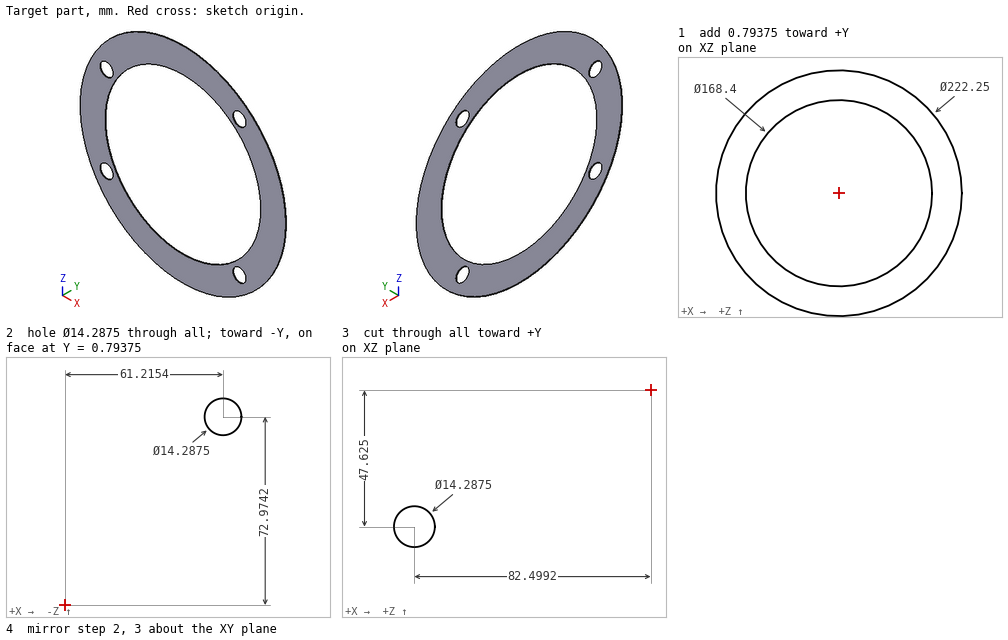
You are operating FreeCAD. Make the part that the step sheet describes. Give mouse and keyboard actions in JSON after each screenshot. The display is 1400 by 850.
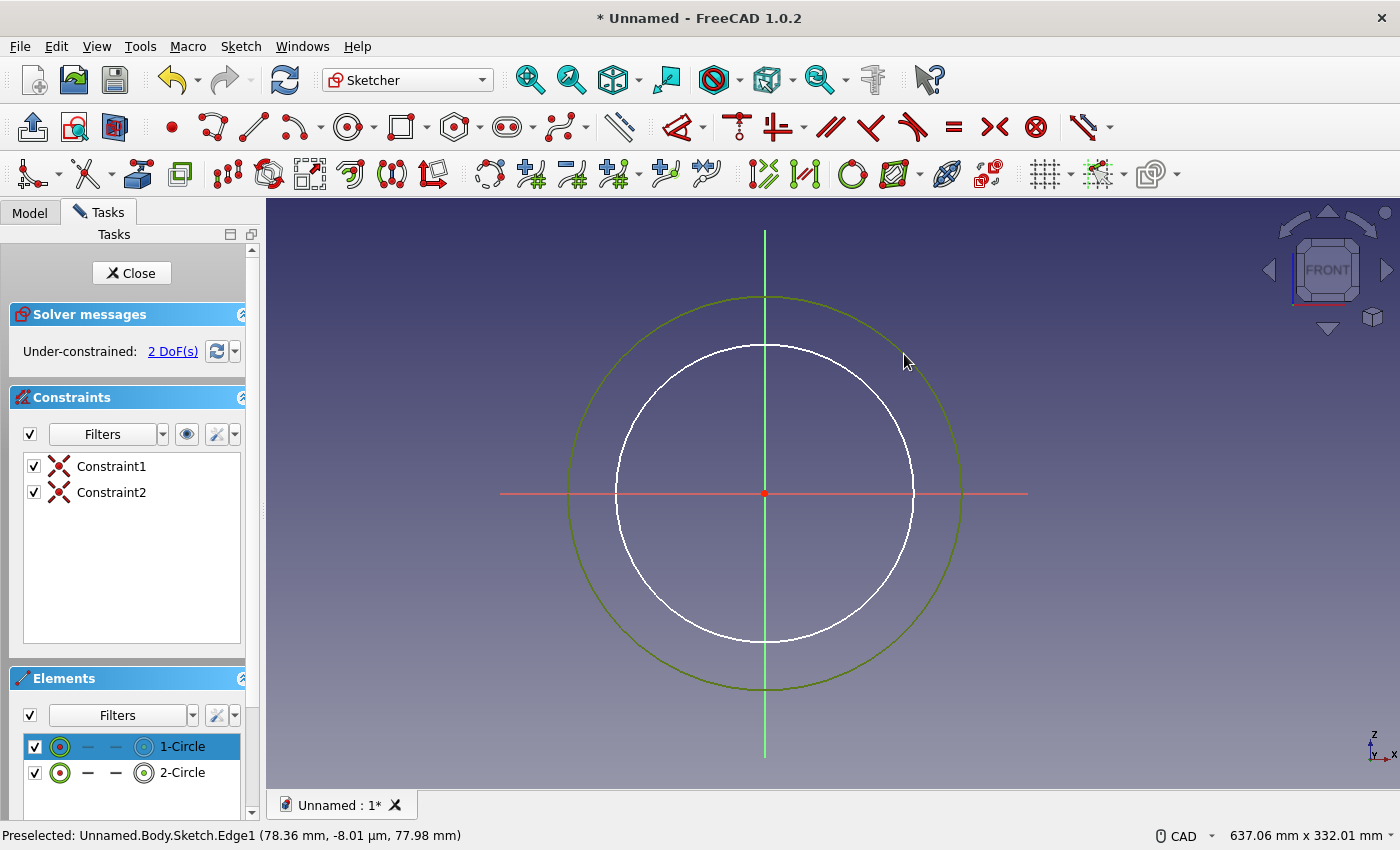
{"action": "left_click", "coordinate": [702, 128]}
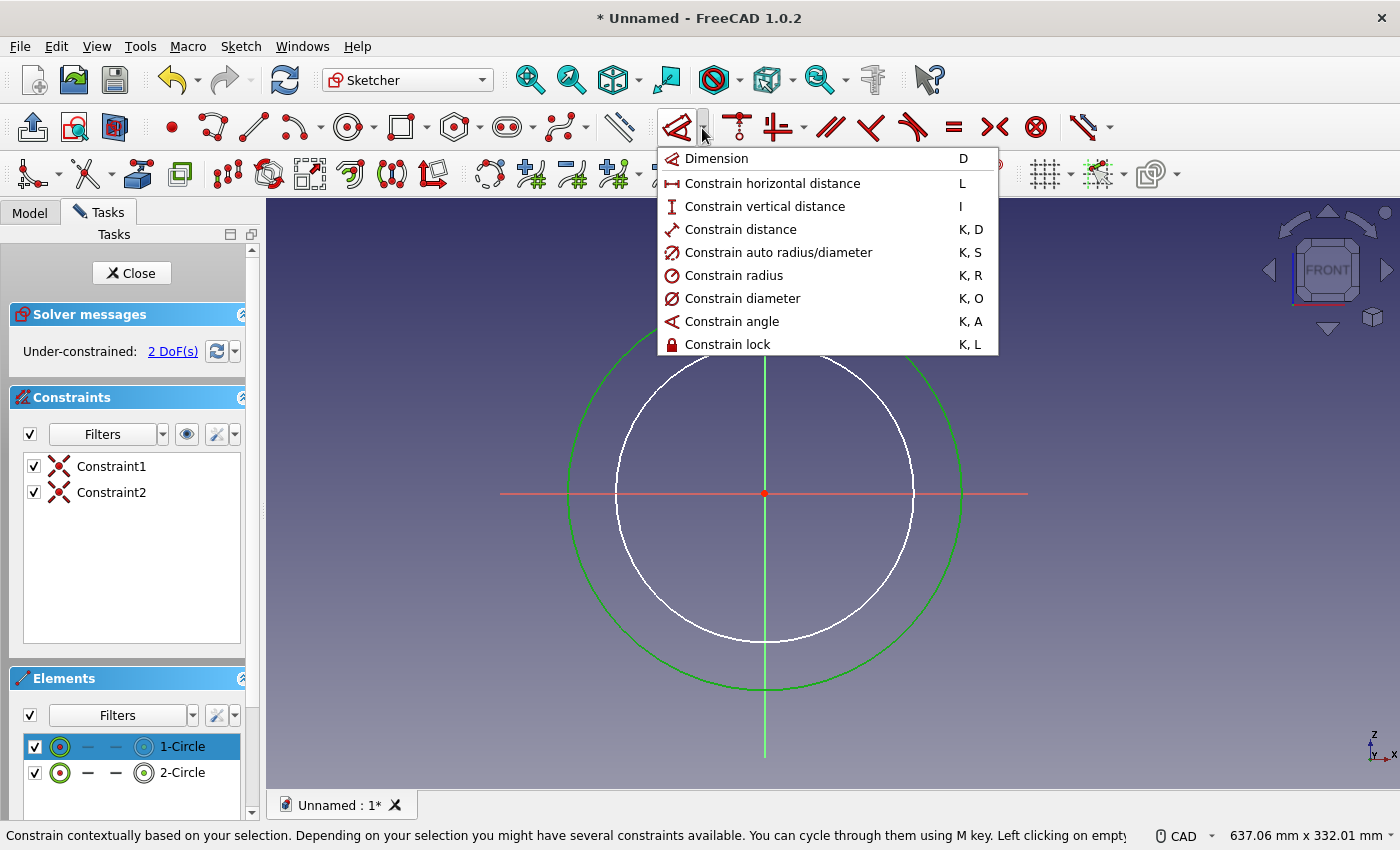
{"action": "left_click", "coordinate": [828, 298]}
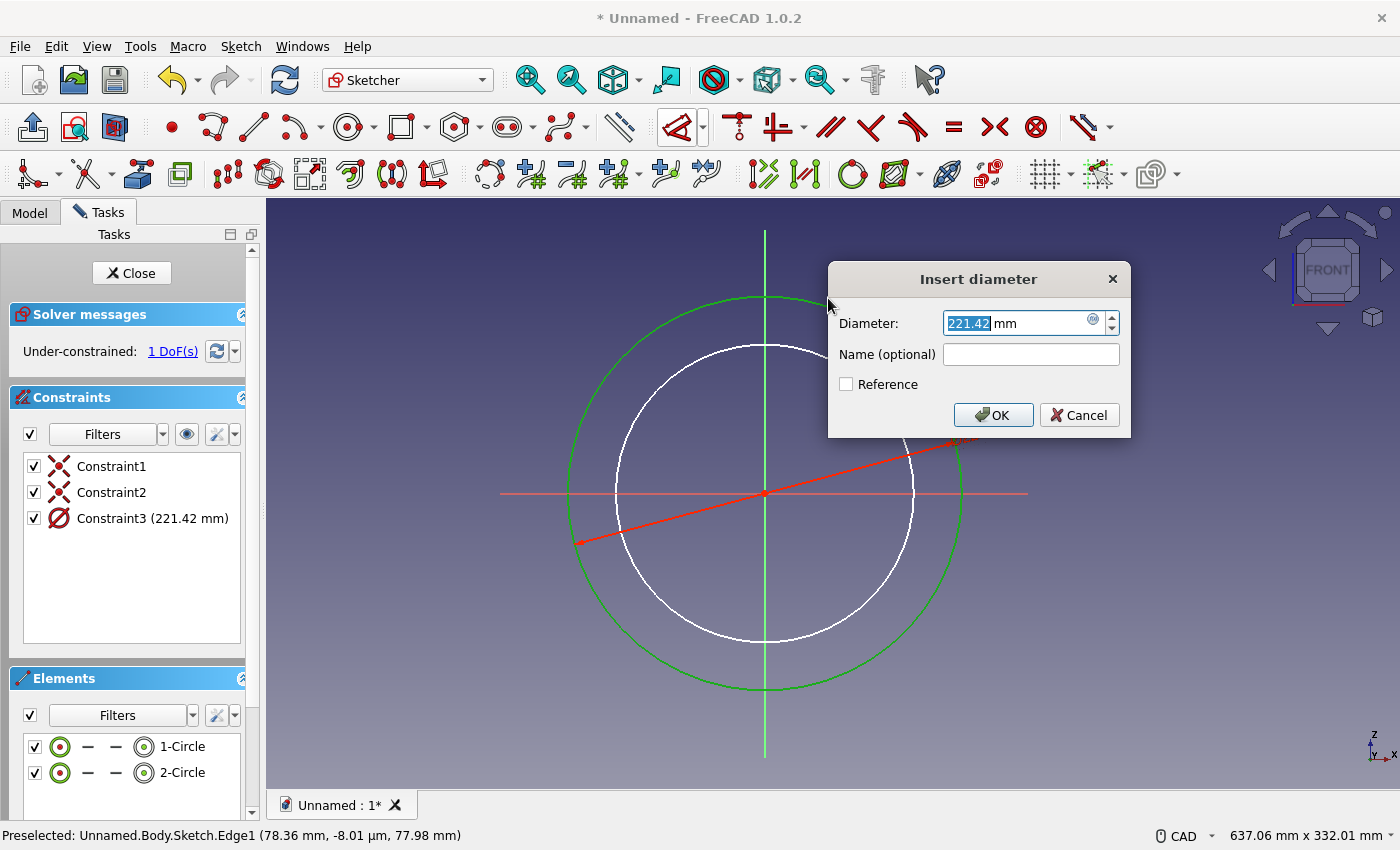
{"action": "type", "text": "222.25"}
{"action": "key", "text": "Return"}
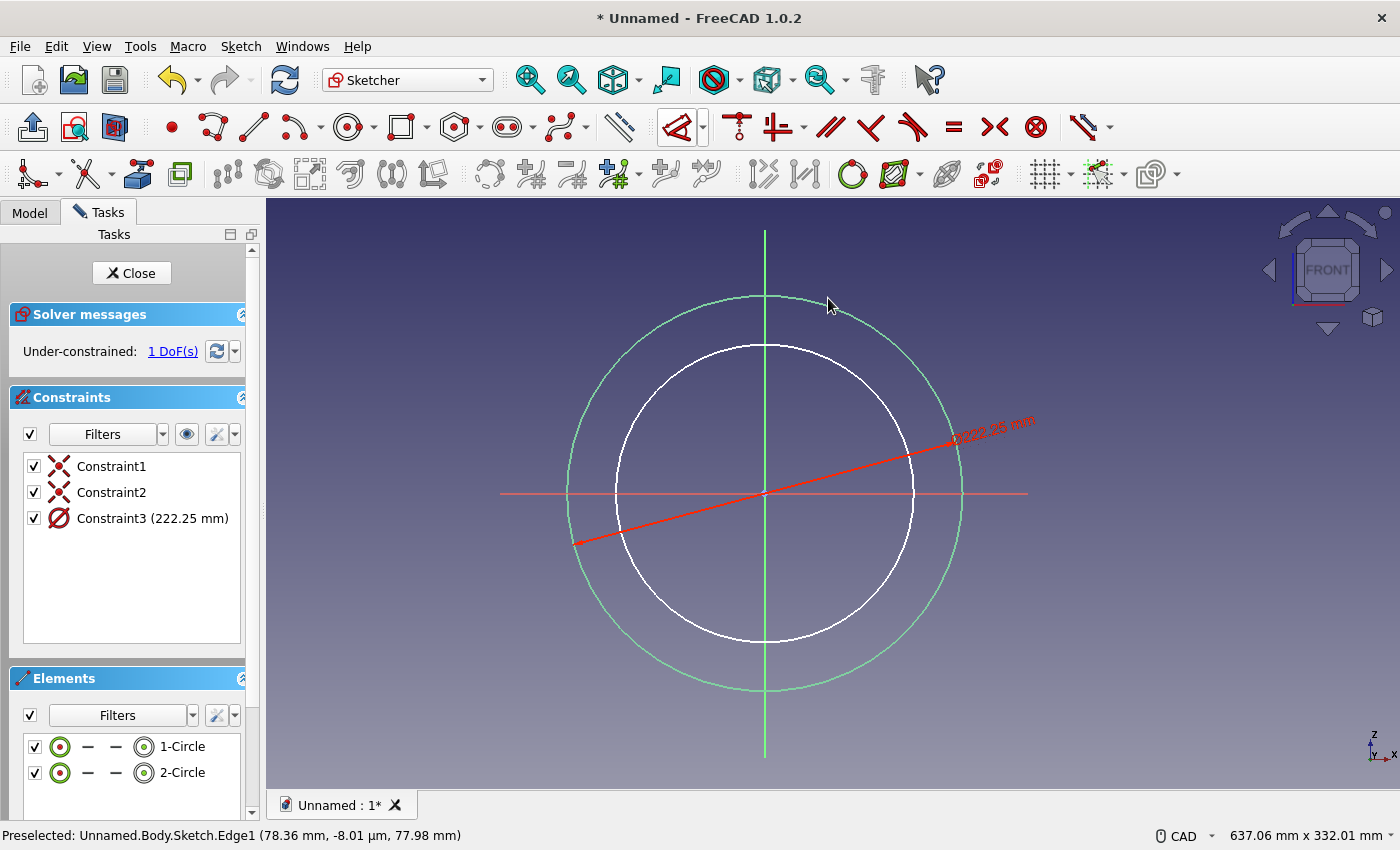
{"action": "left_click", "coordinate": [870, 388]}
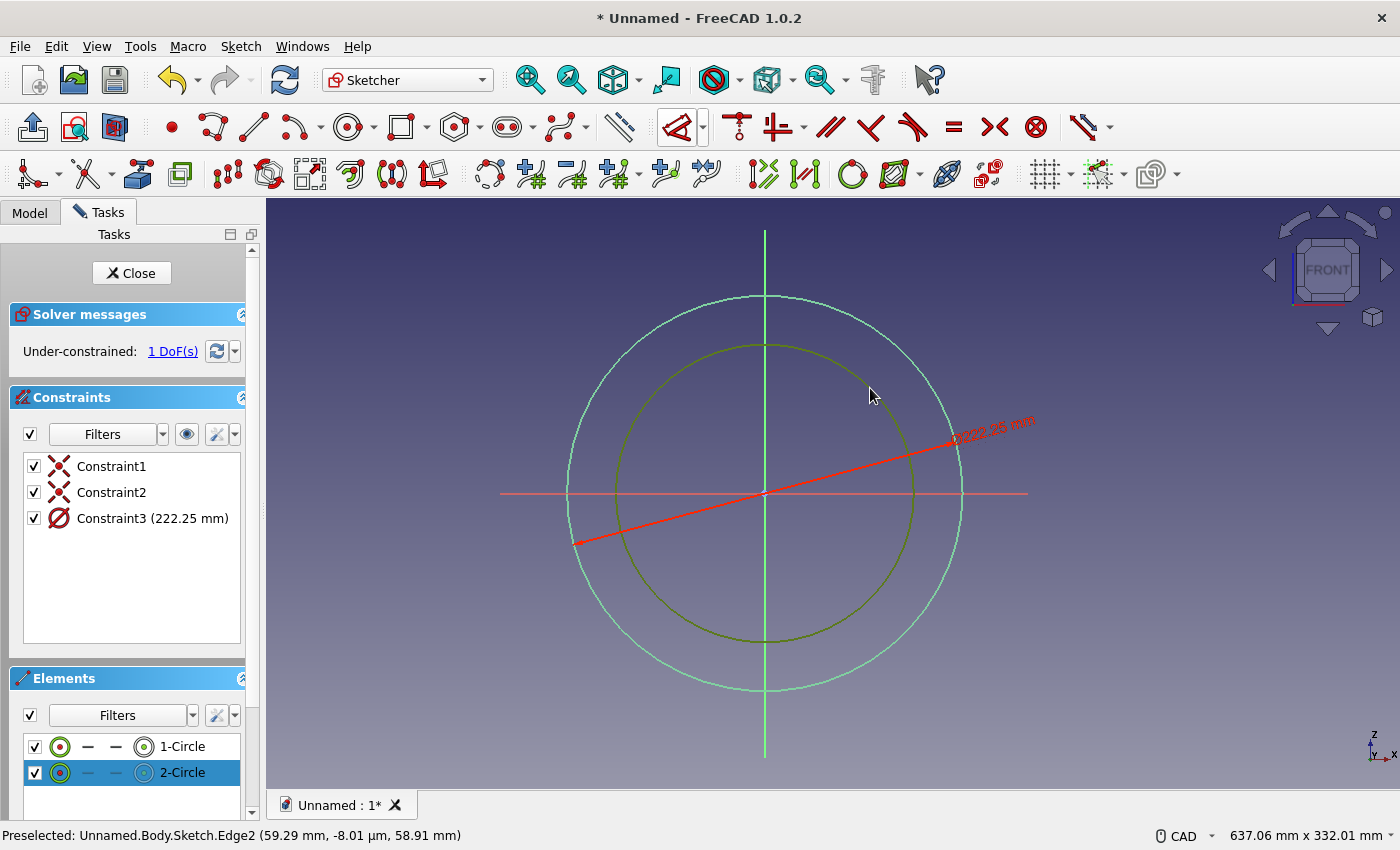
{"action": "key", "text": "k o"}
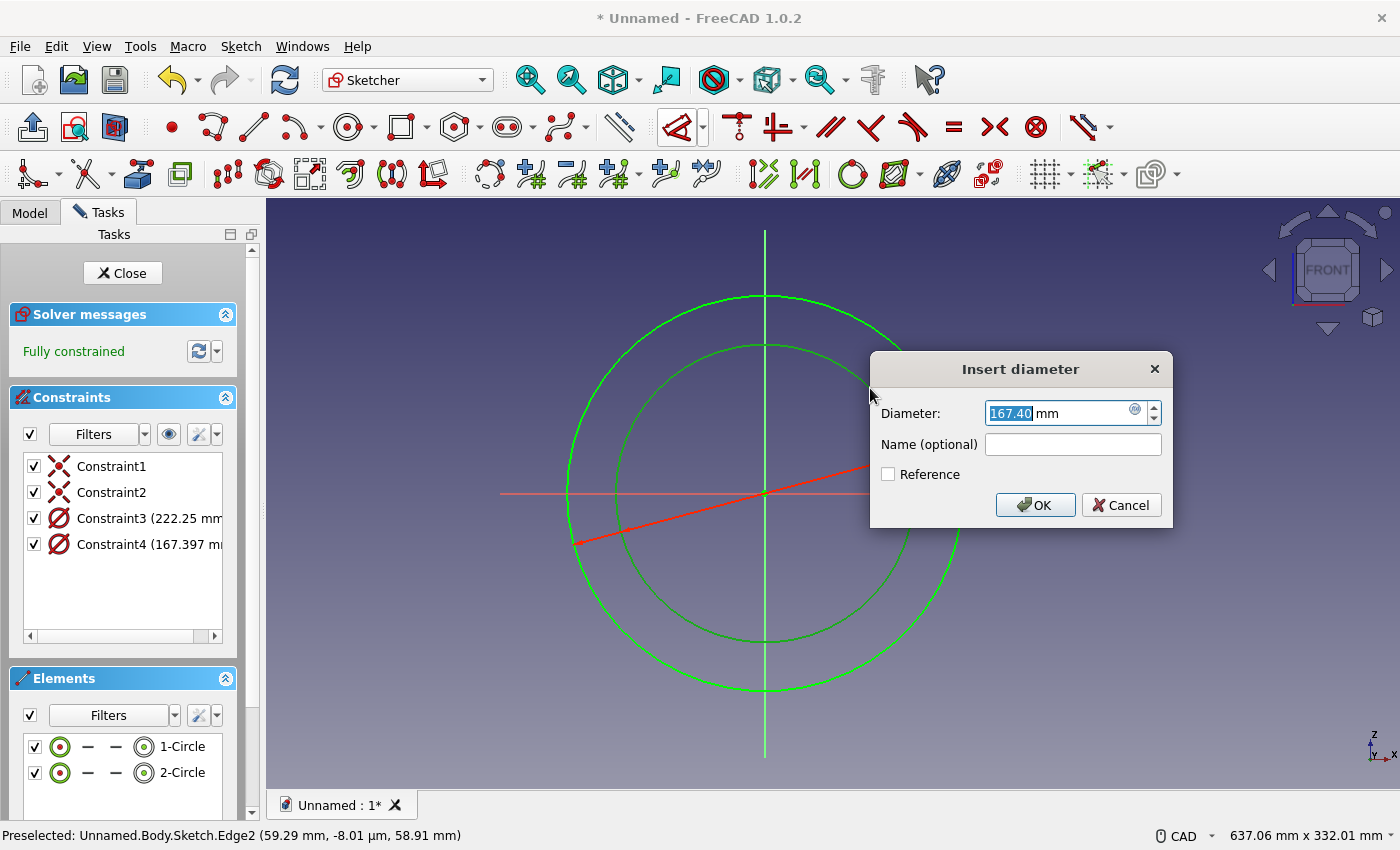
{"action": "type", "text": "168.4"}
{"action": "key", "text": "Return"}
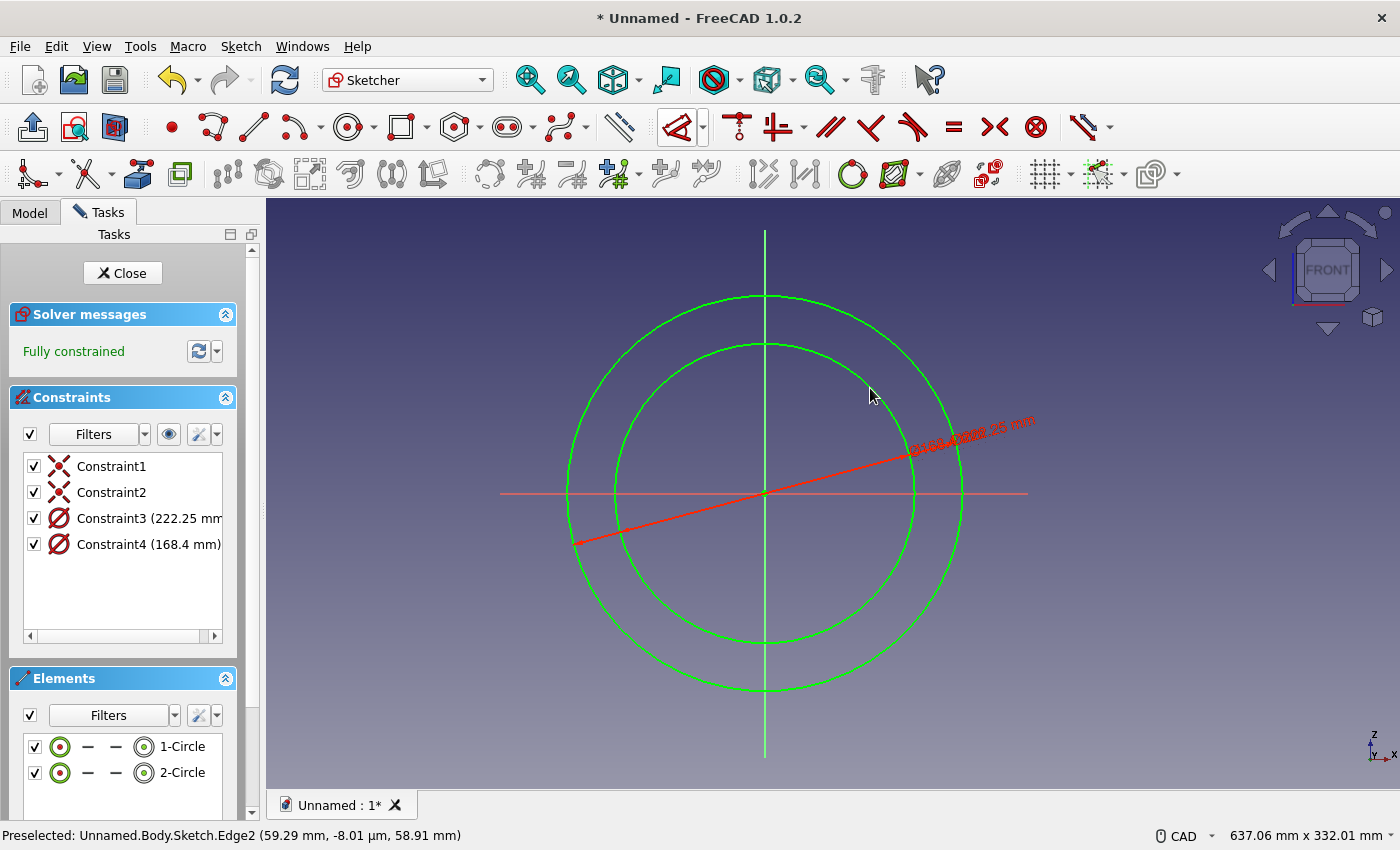
{"action": "left_click", "coordinate": [123, 273]}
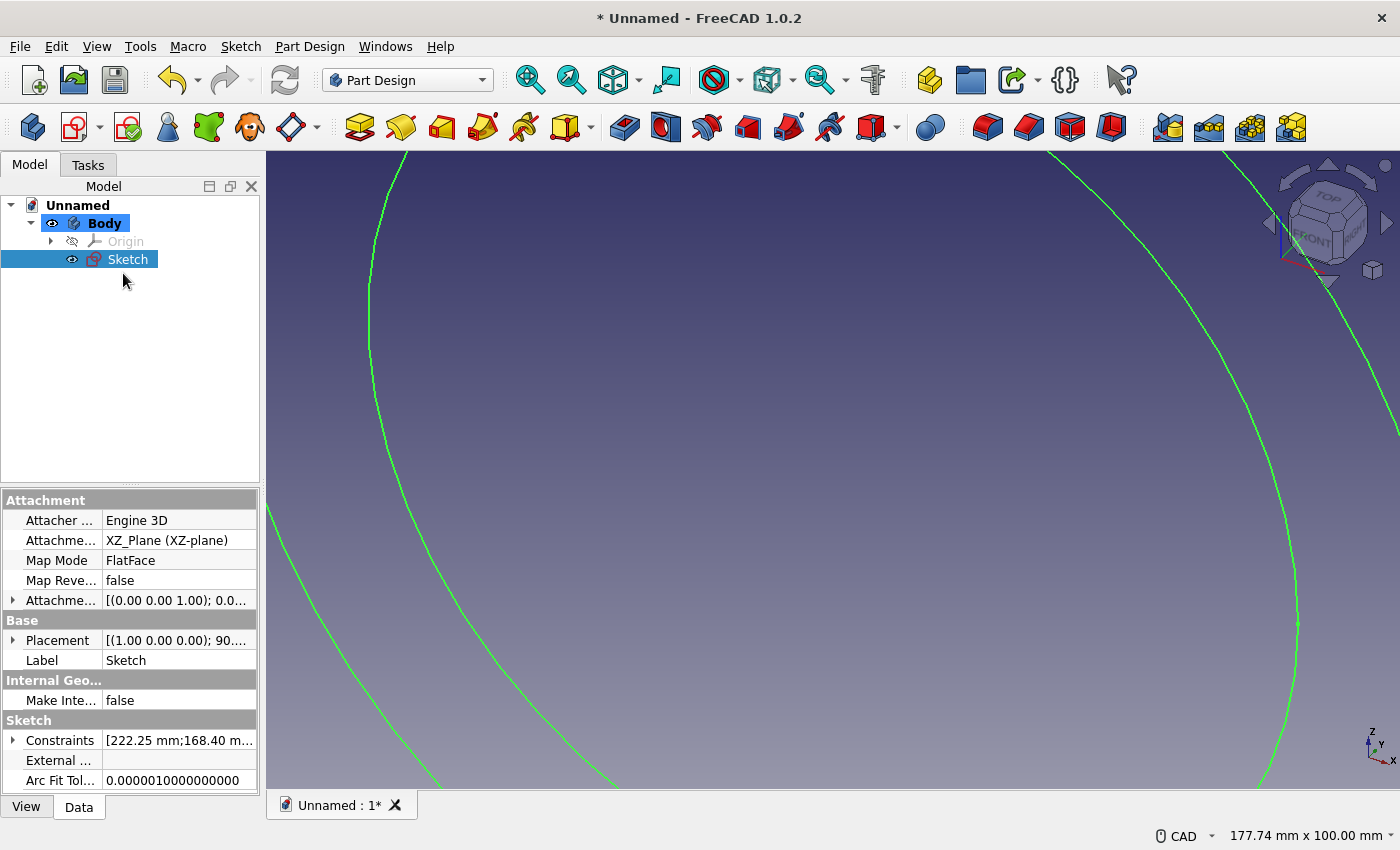
{"action": "left_click", "coordinate": [360, 128]}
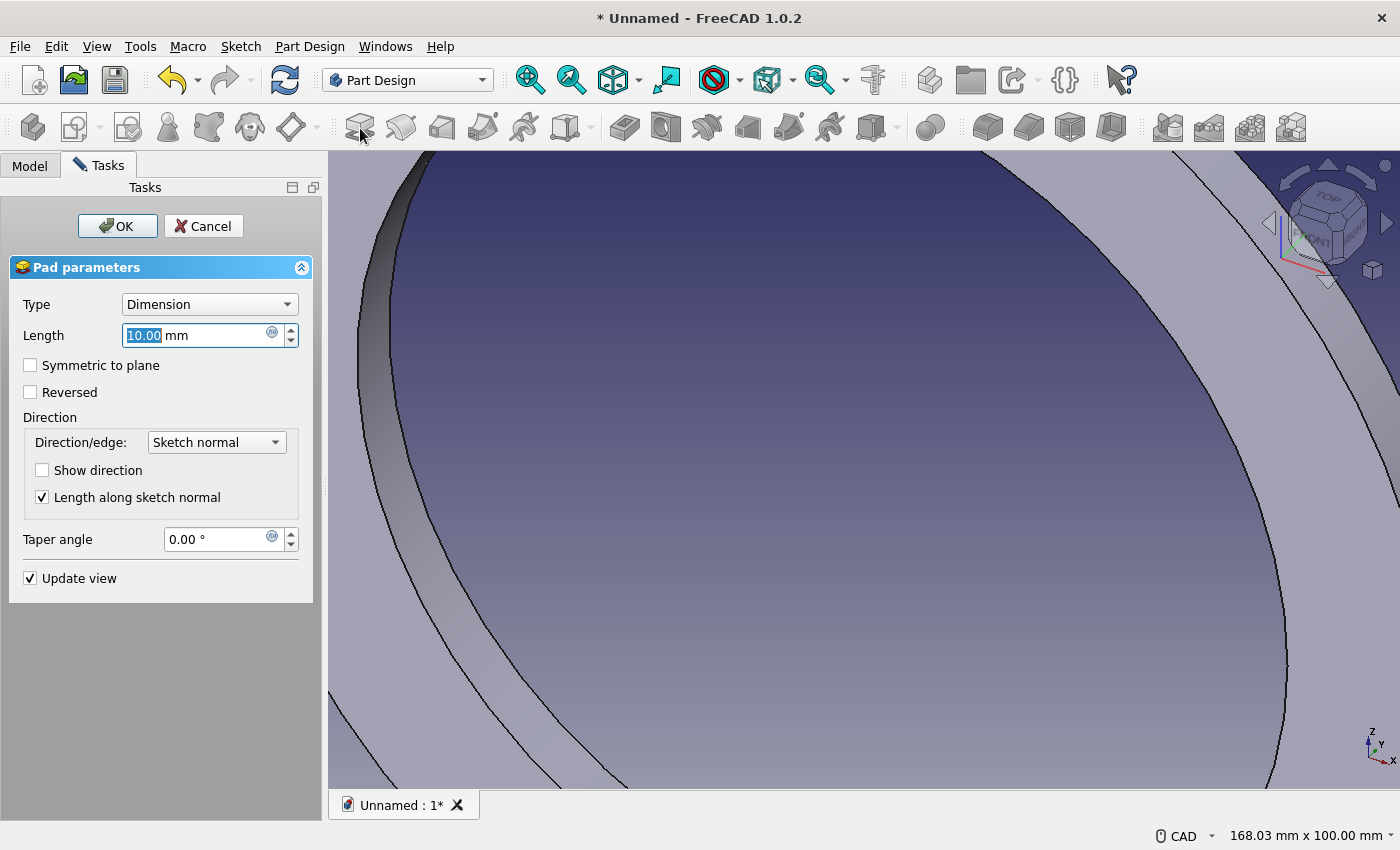
{"action": "type", "text": "0.79375"}
{"action": "key", "text": "Tab"}